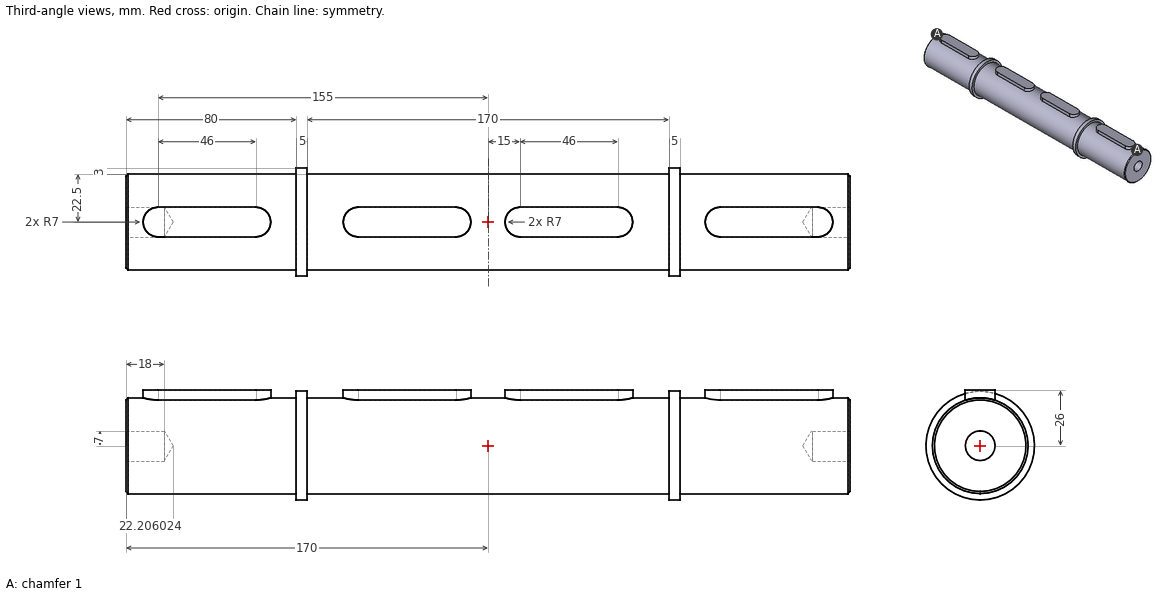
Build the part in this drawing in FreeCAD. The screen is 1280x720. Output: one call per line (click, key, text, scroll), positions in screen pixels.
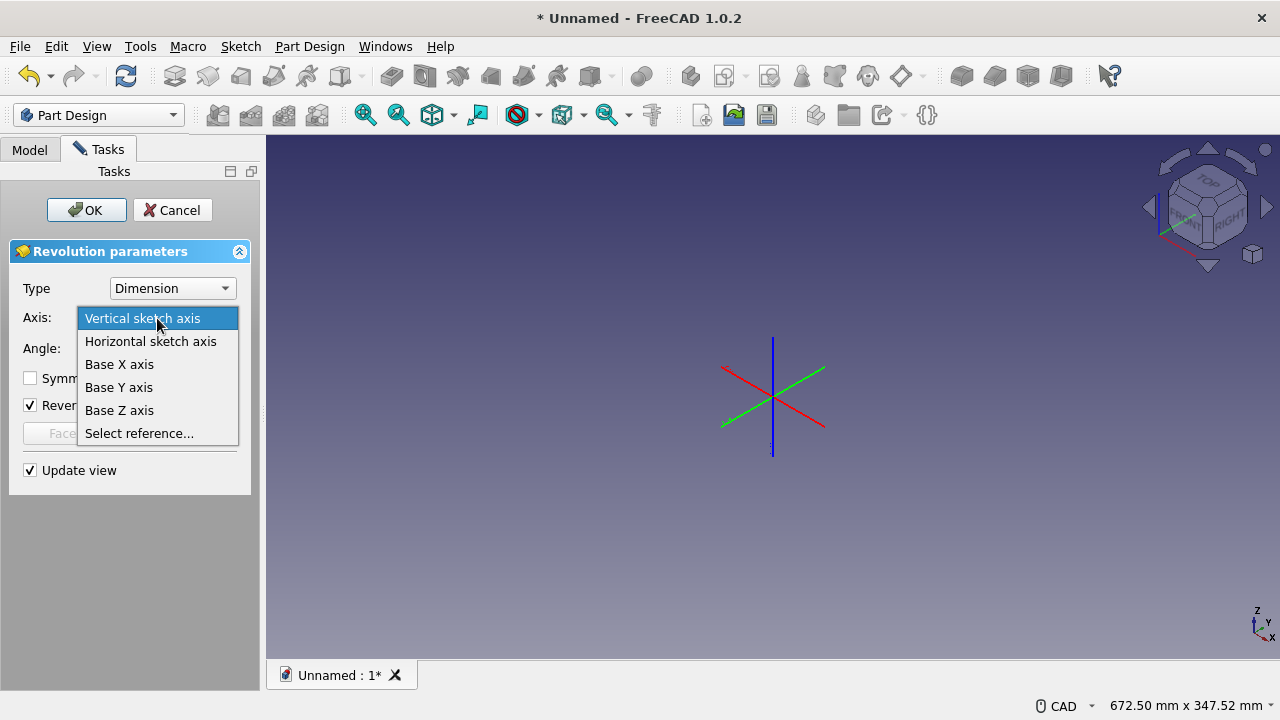
click(156, 342)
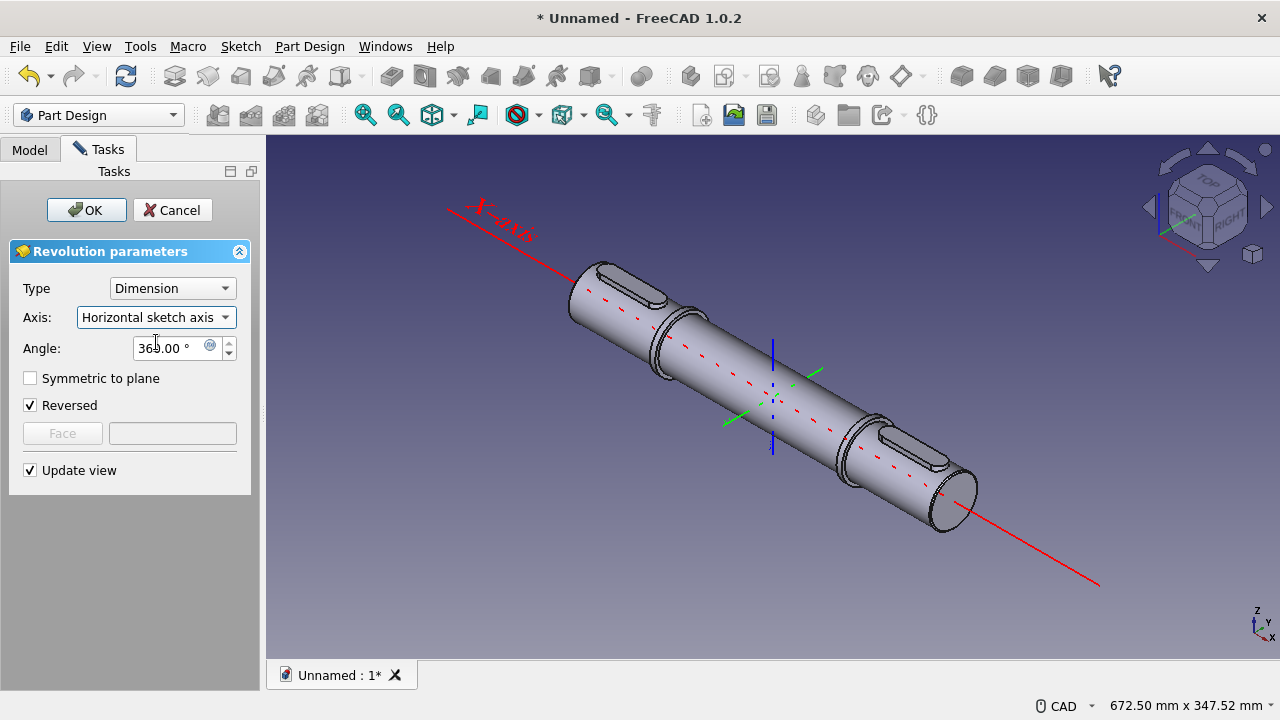
click(87, 210)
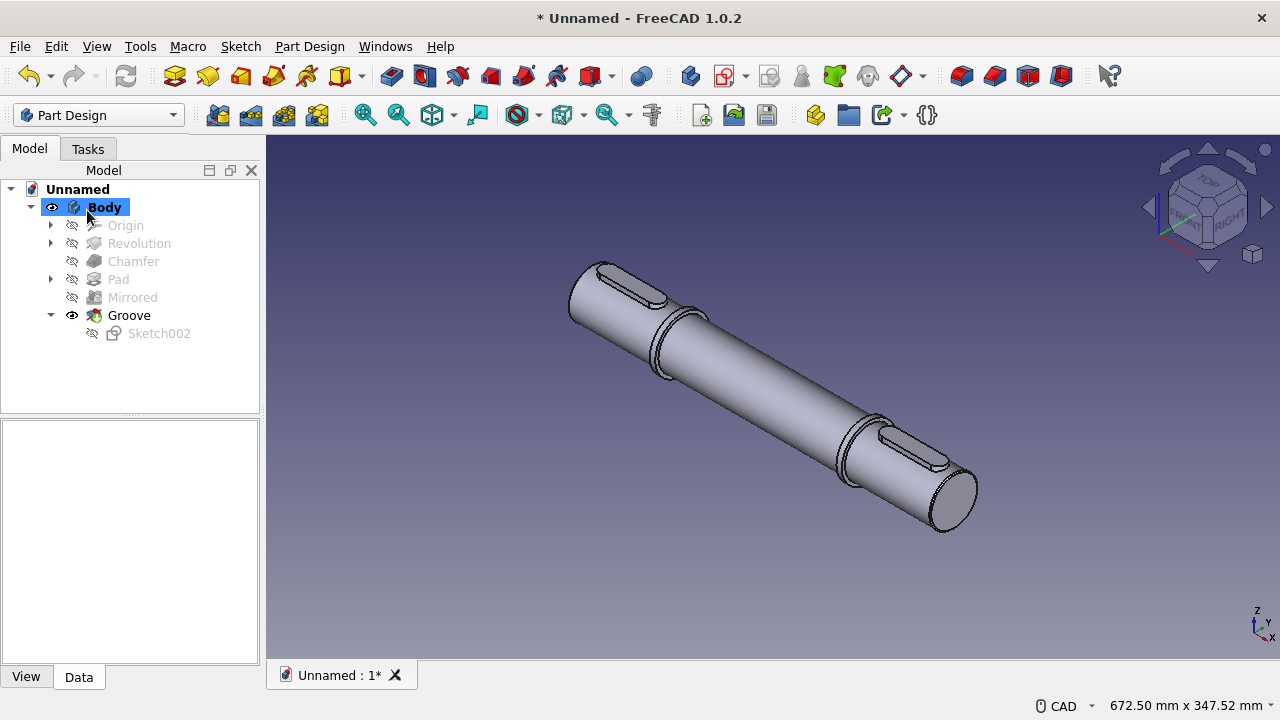
click(117, 315)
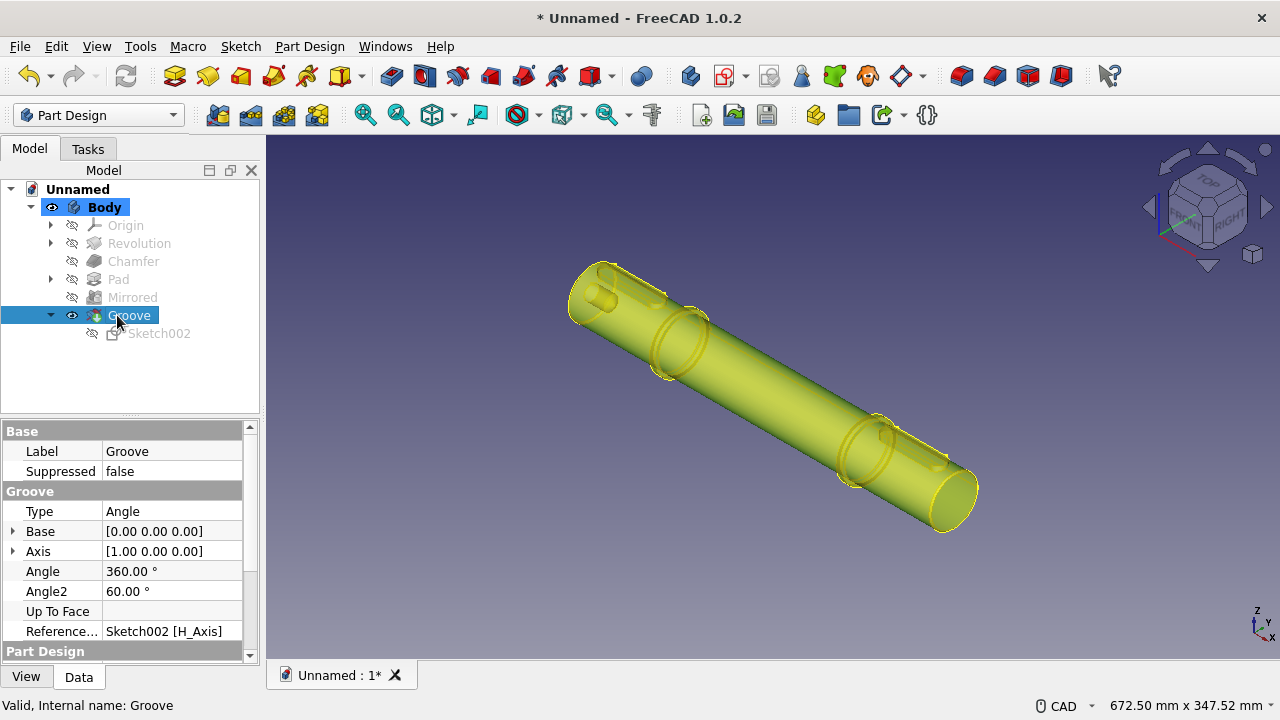
click(218, 116)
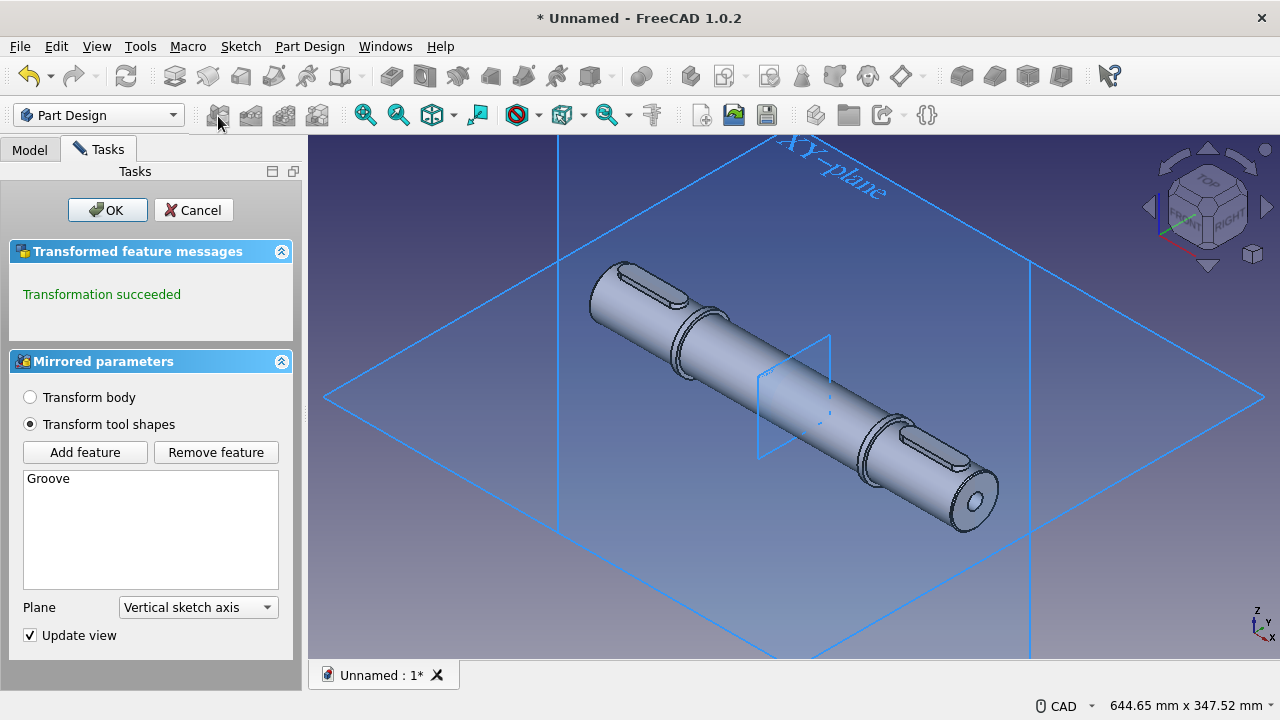
click(199, 608)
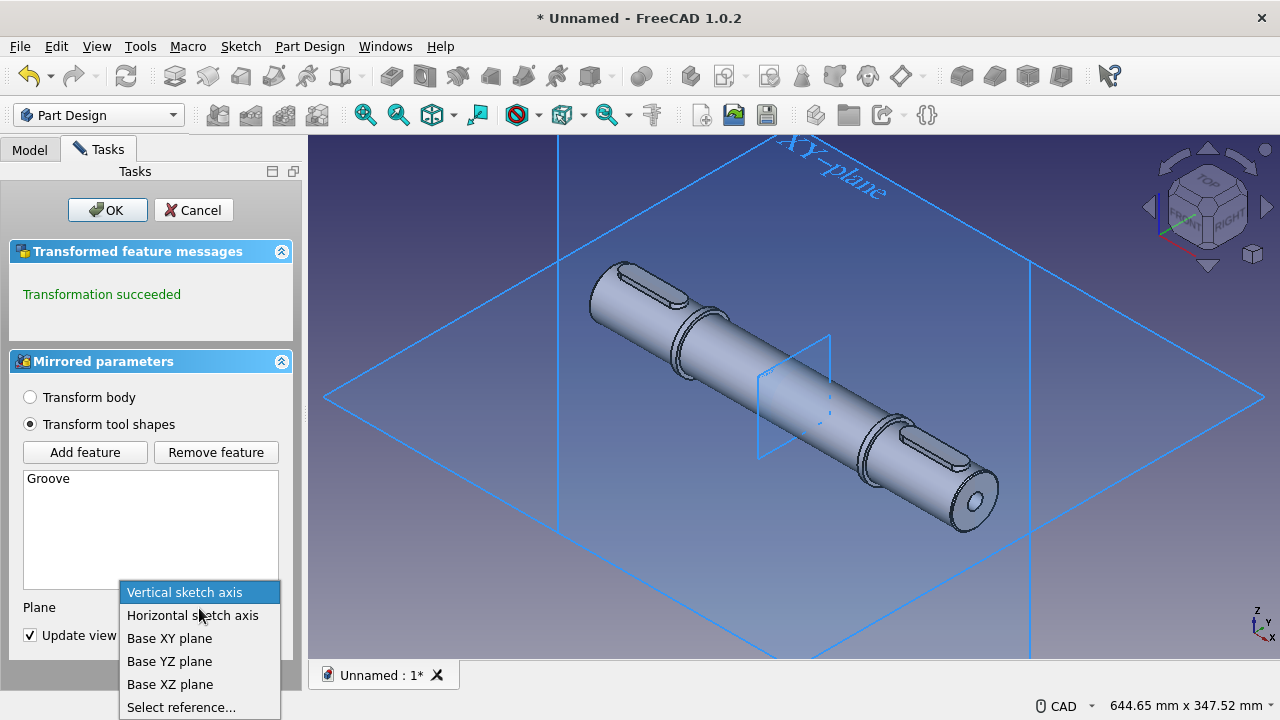
click(198, 662)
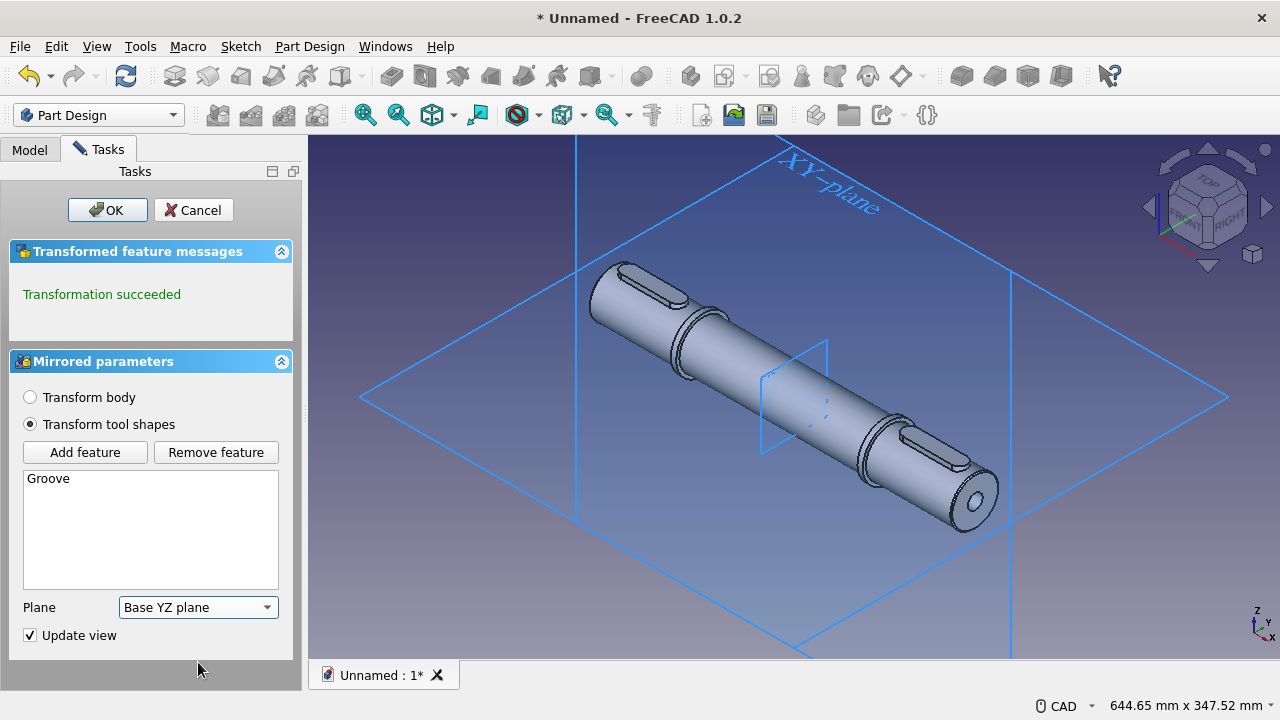
click(108, 210)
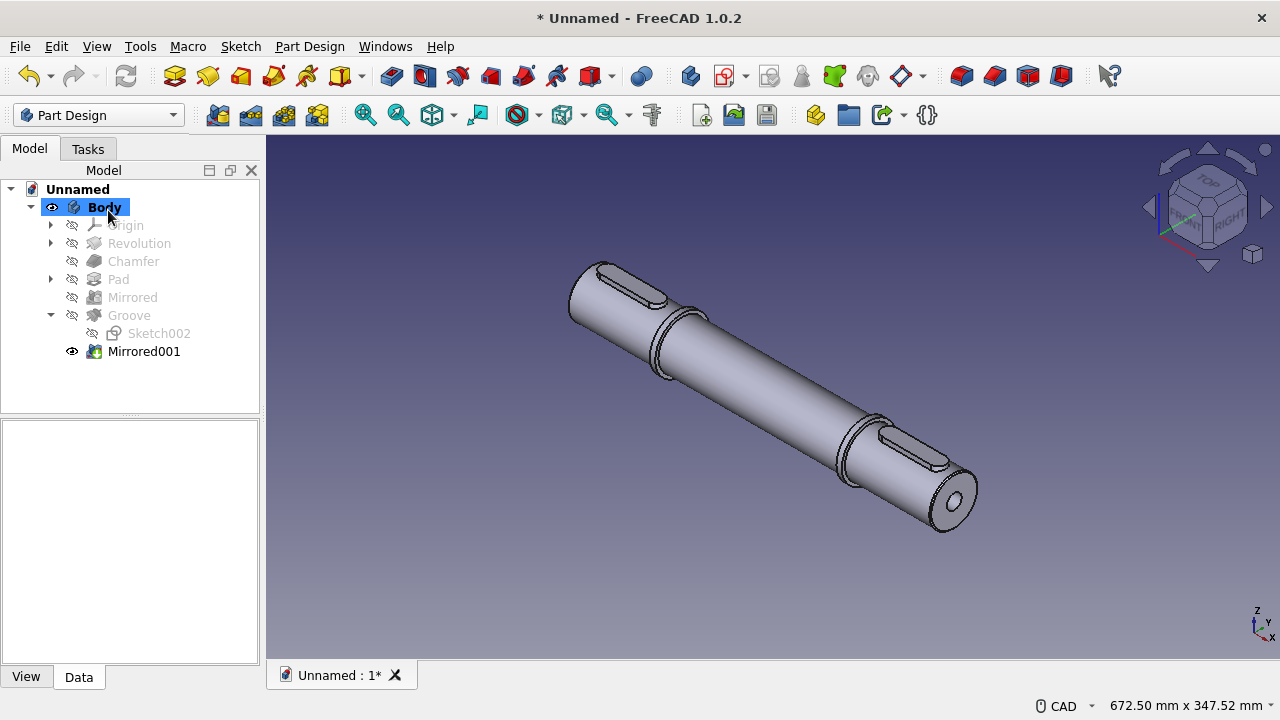
click(51, 225)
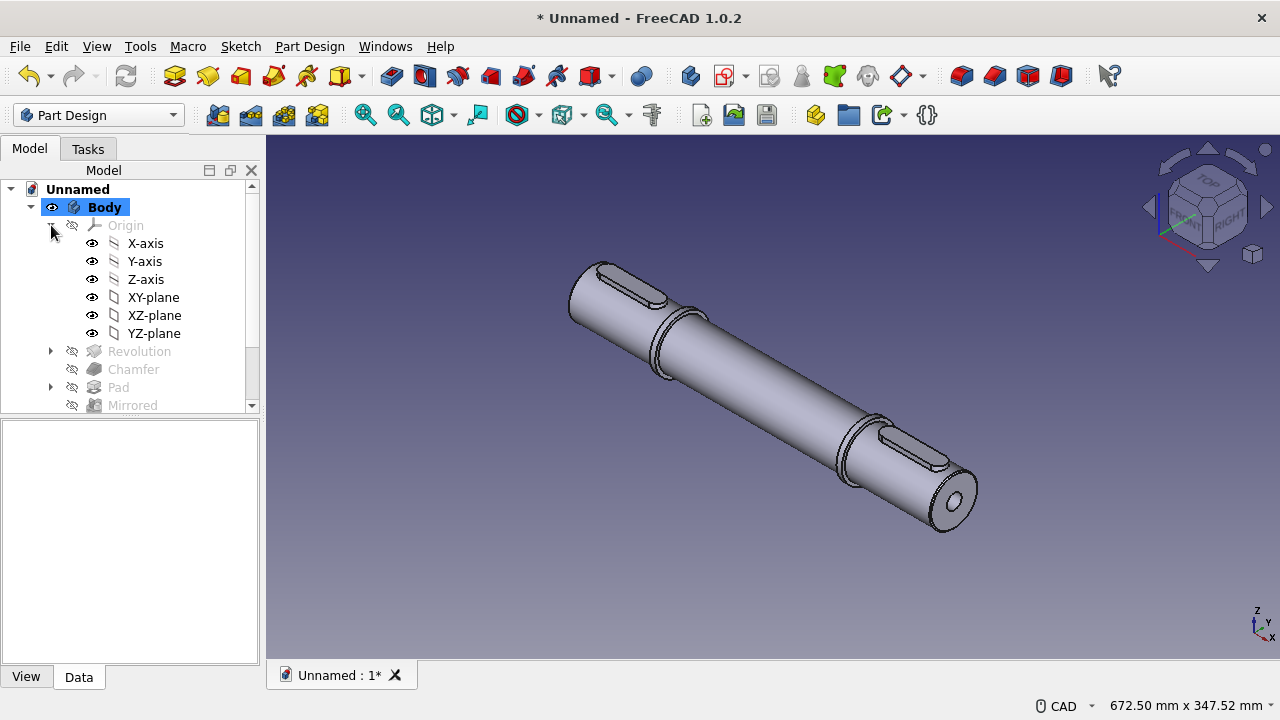
click(137, 333)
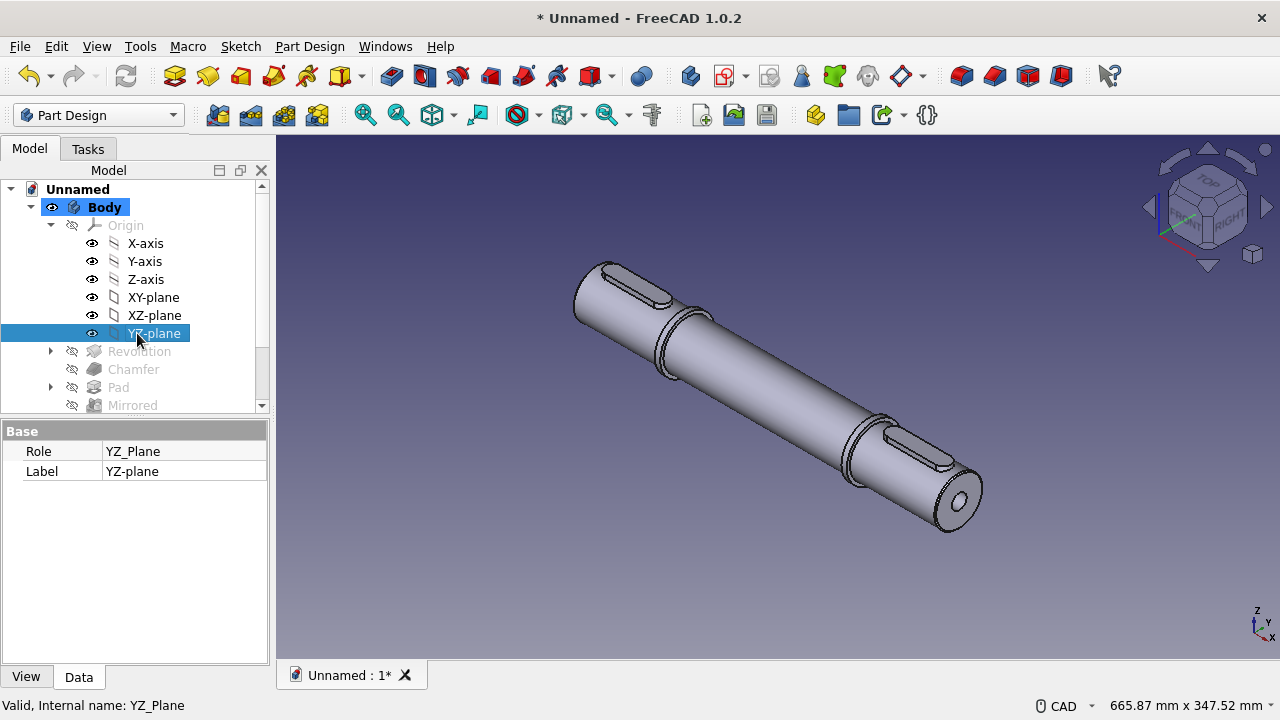
click(900, 76)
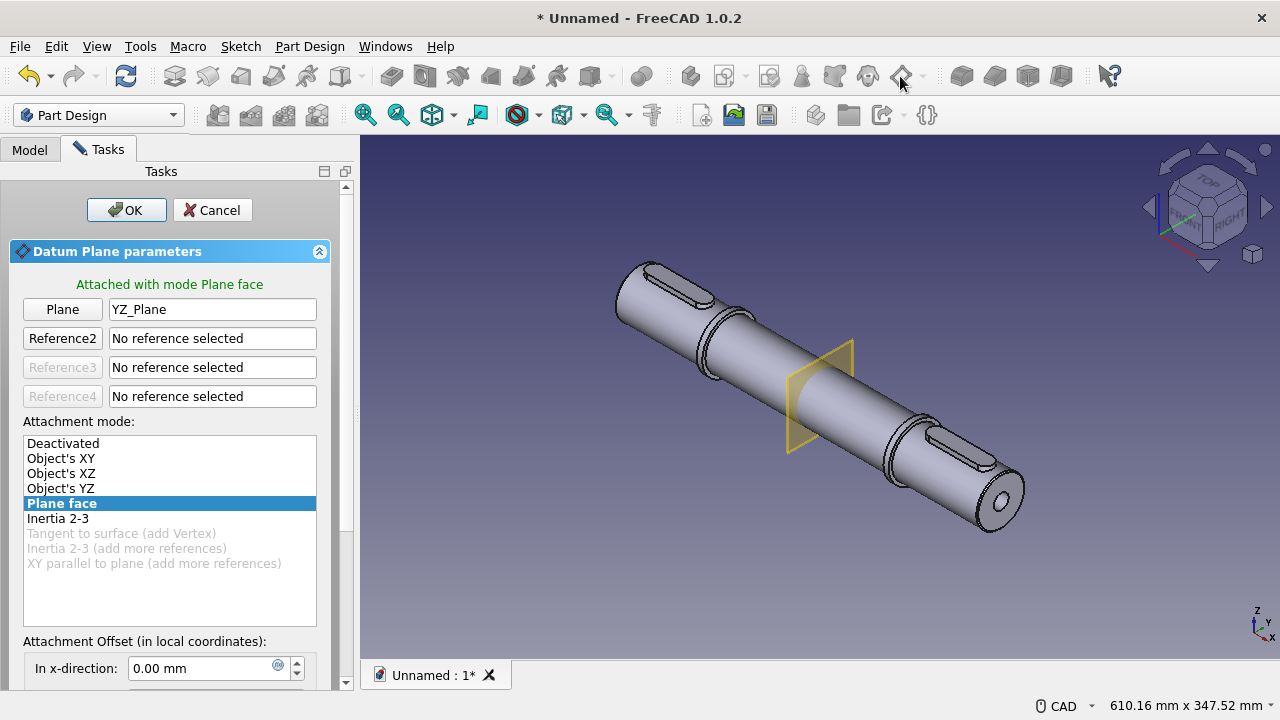
scroll(346, 436, down, 2)